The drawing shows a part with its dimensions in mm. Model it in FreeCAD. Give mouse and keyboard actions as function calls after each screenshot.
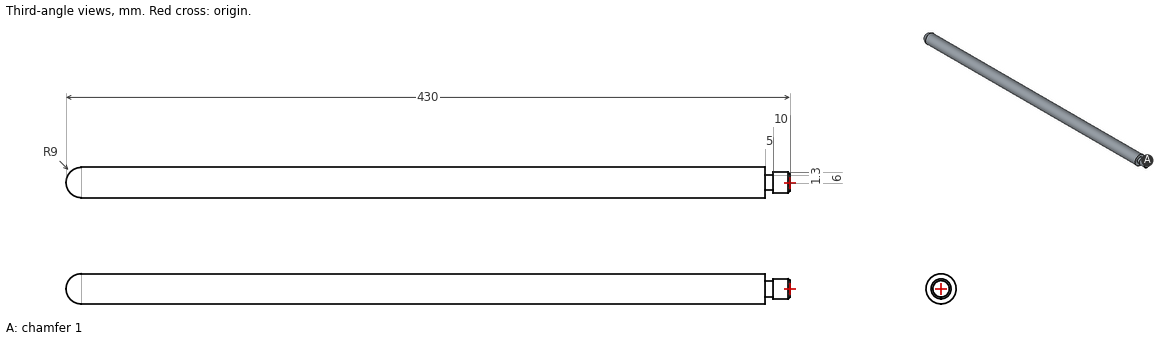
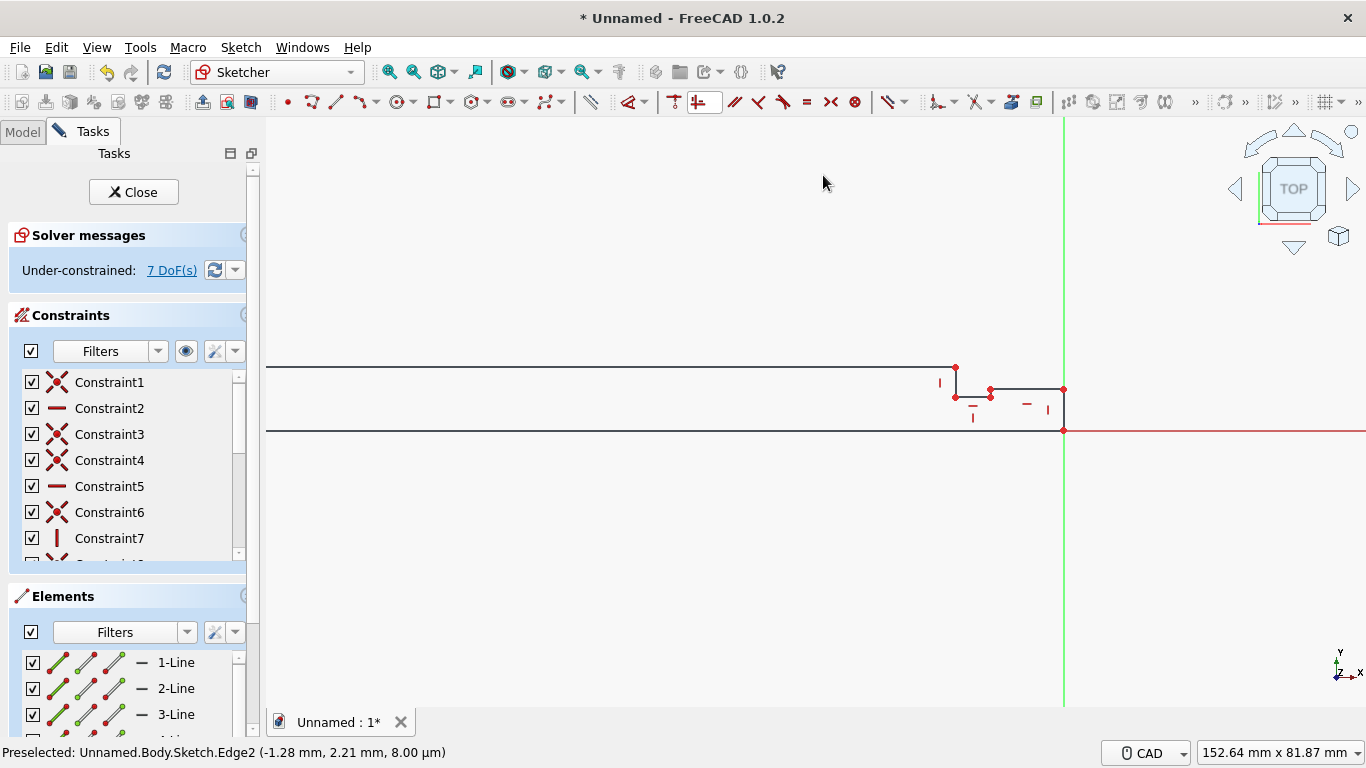
scroll(1059, 415, down, 8)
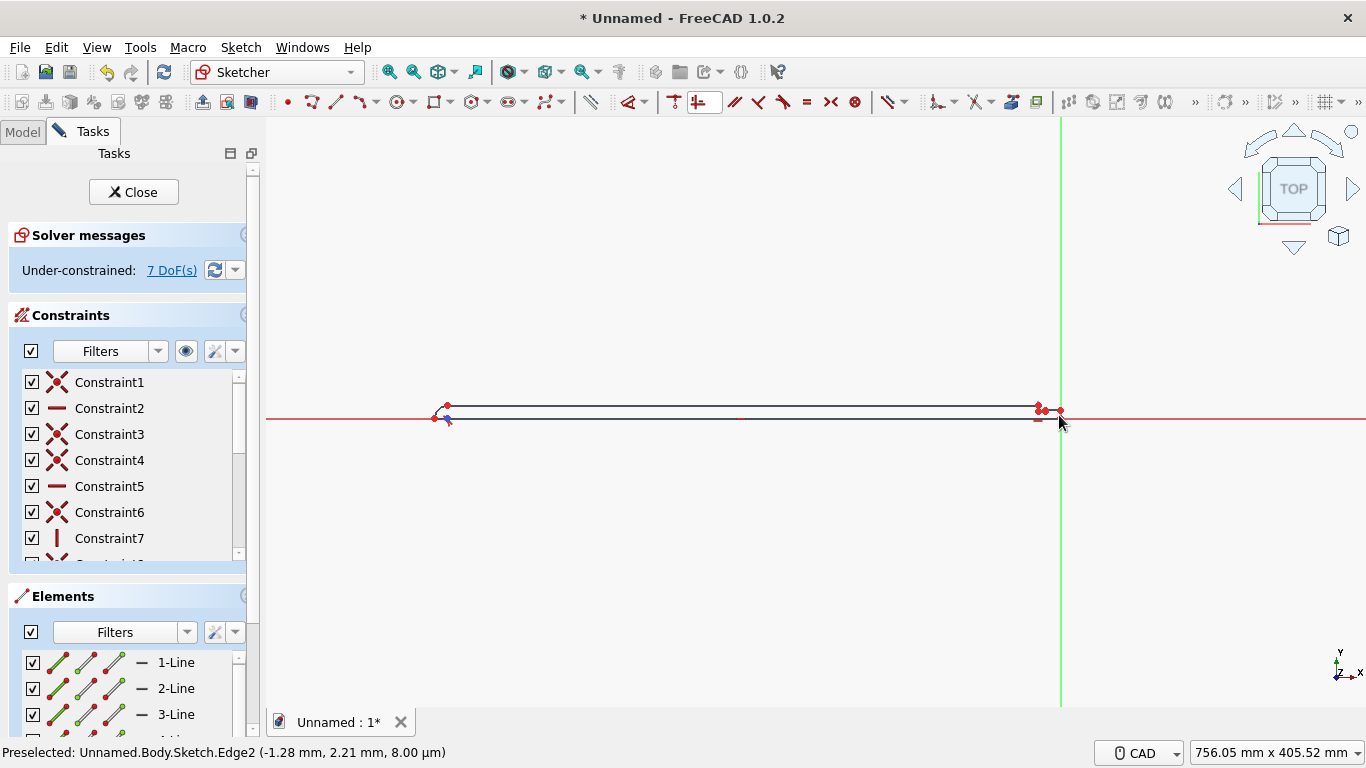
click(448, 419)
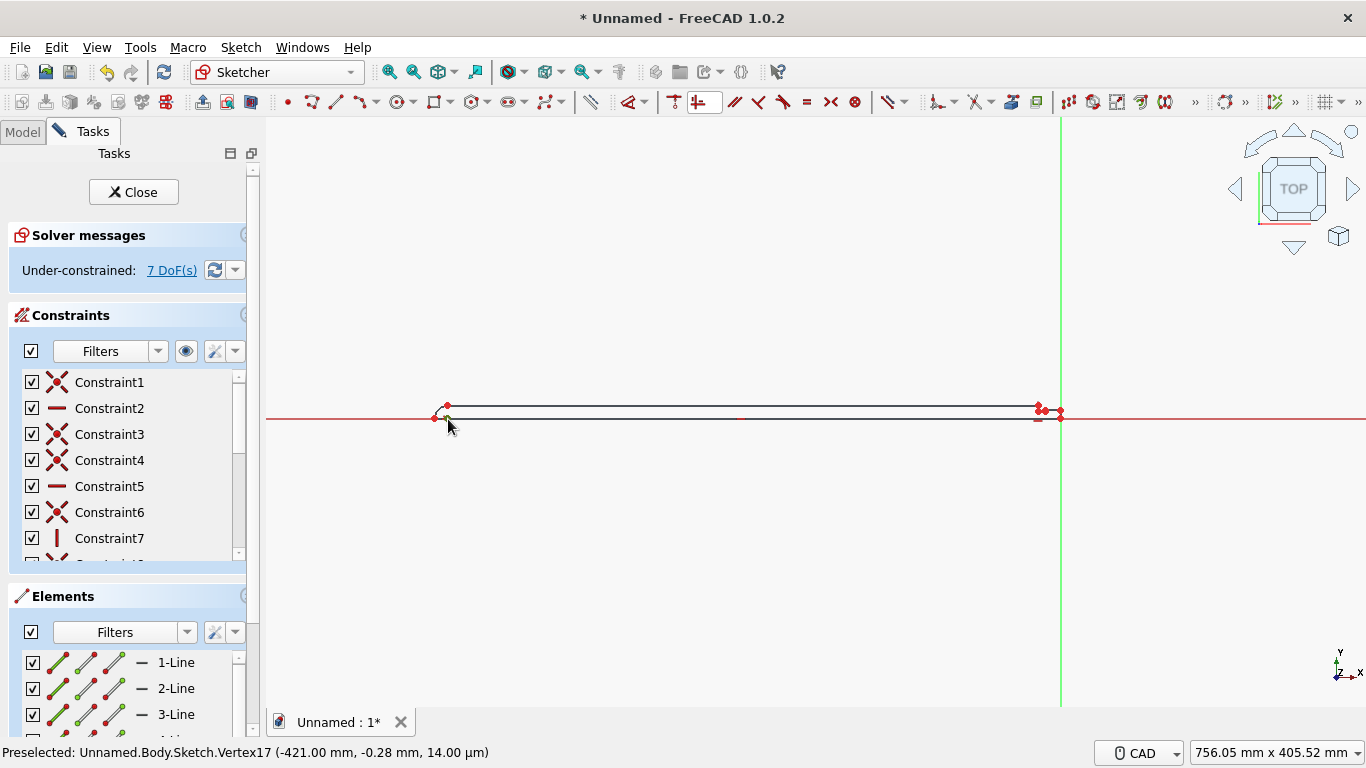
click(359, 419)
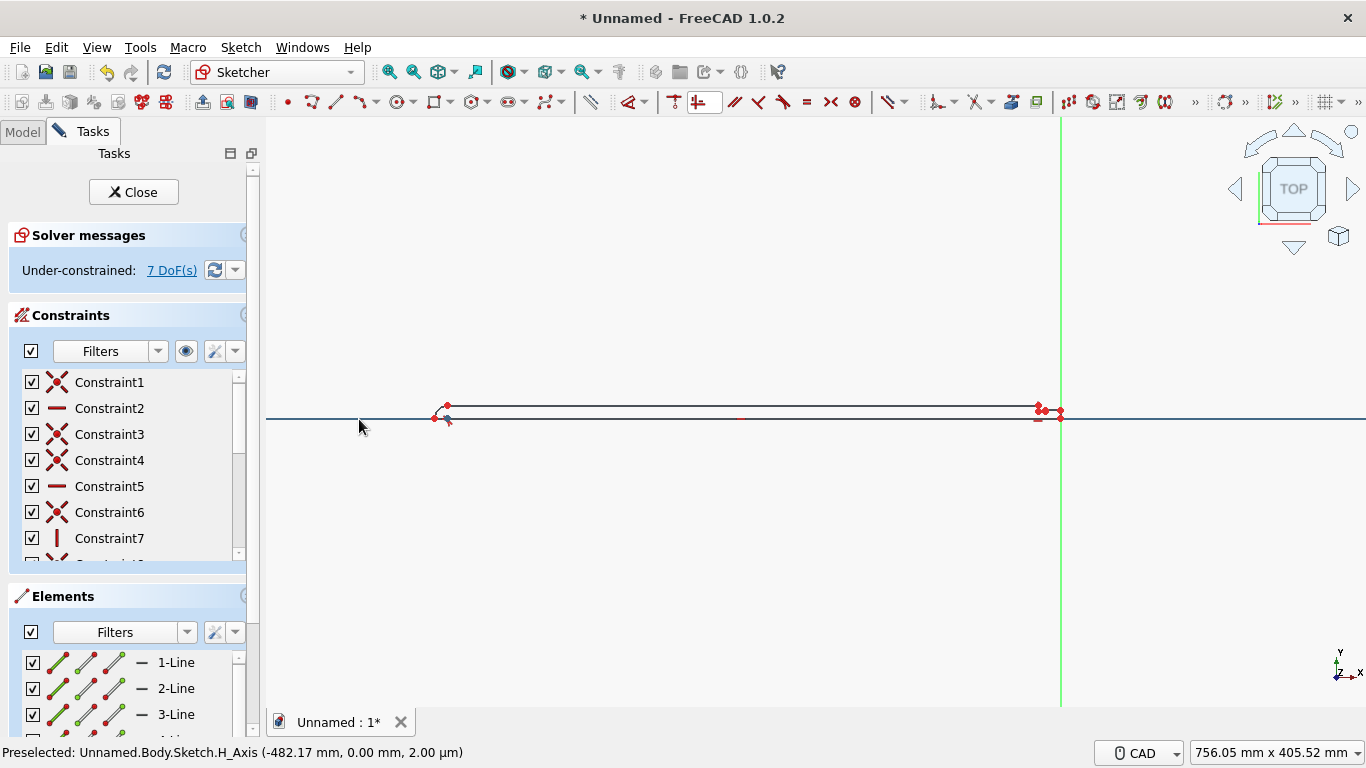
click(674, 102)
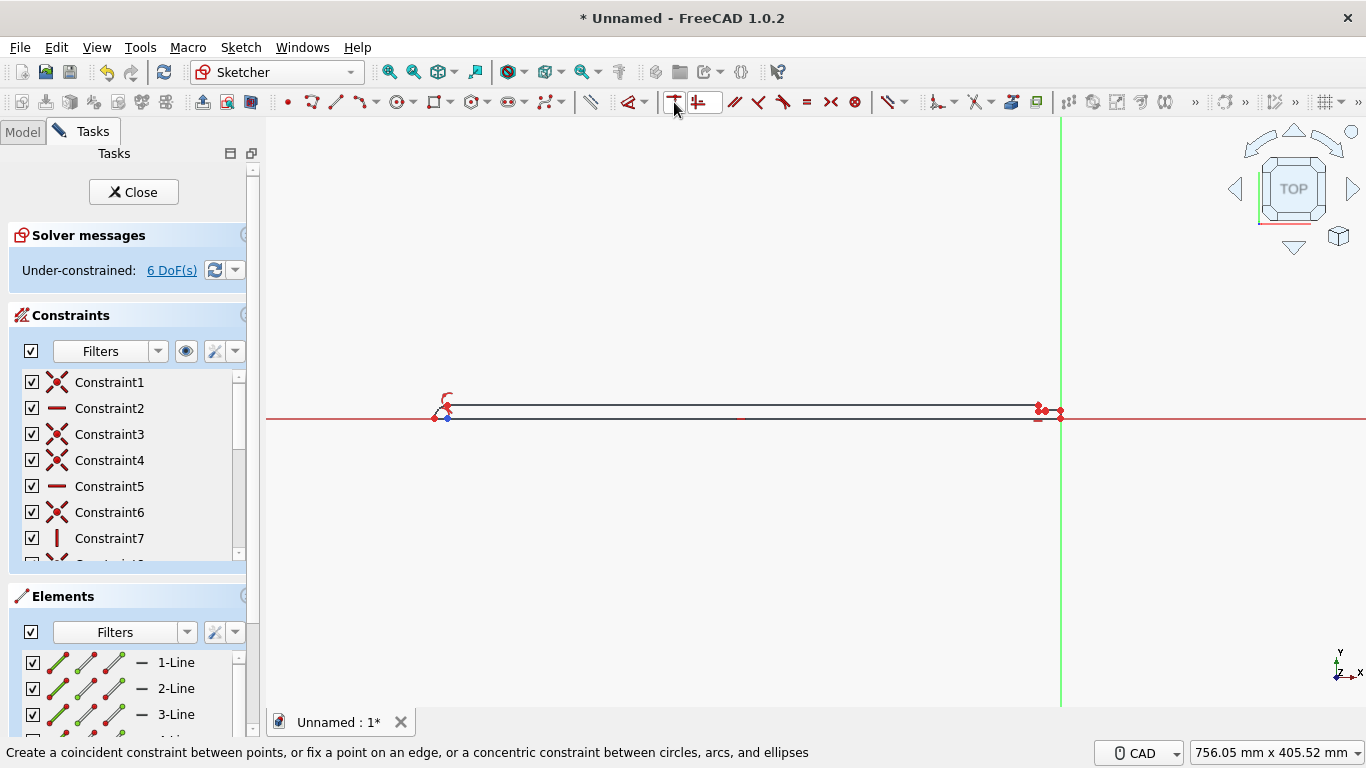
click(628, 102)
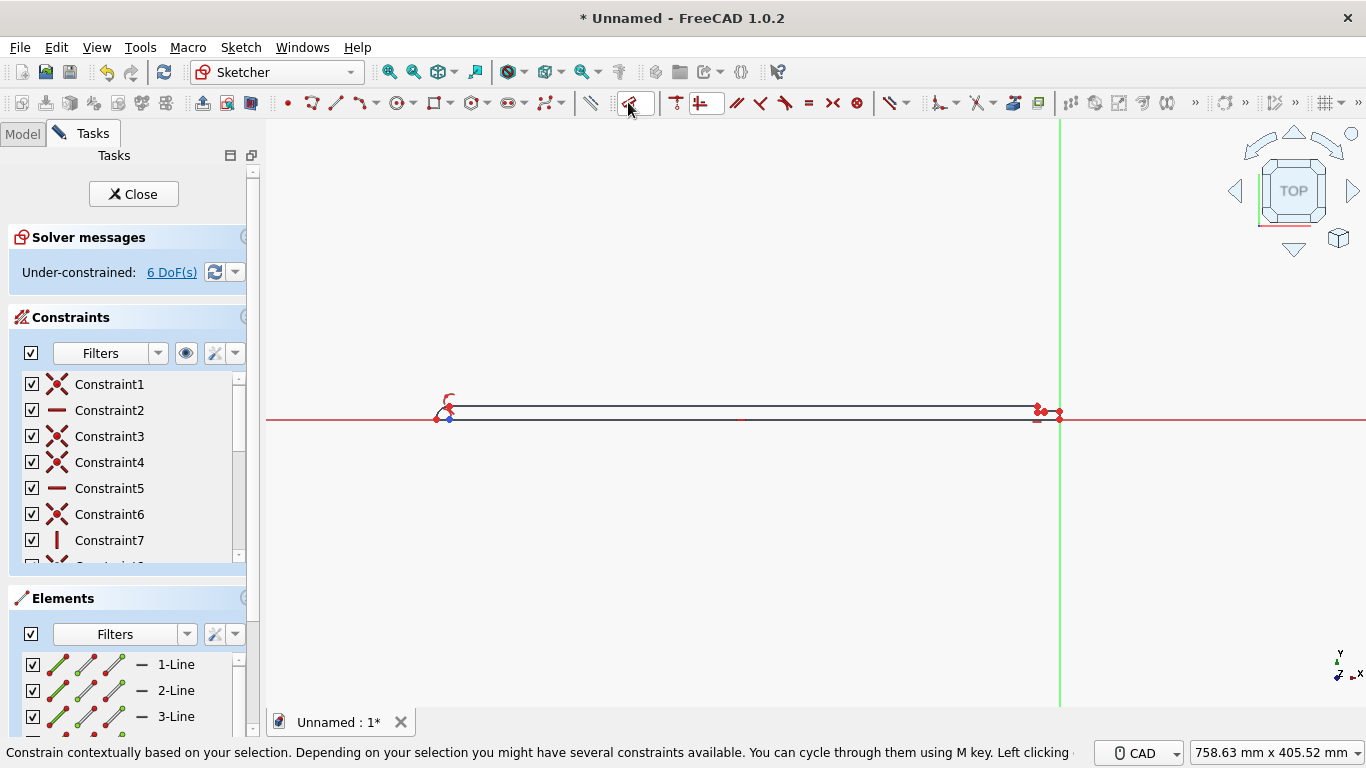
scroll(440, 410, up, 6)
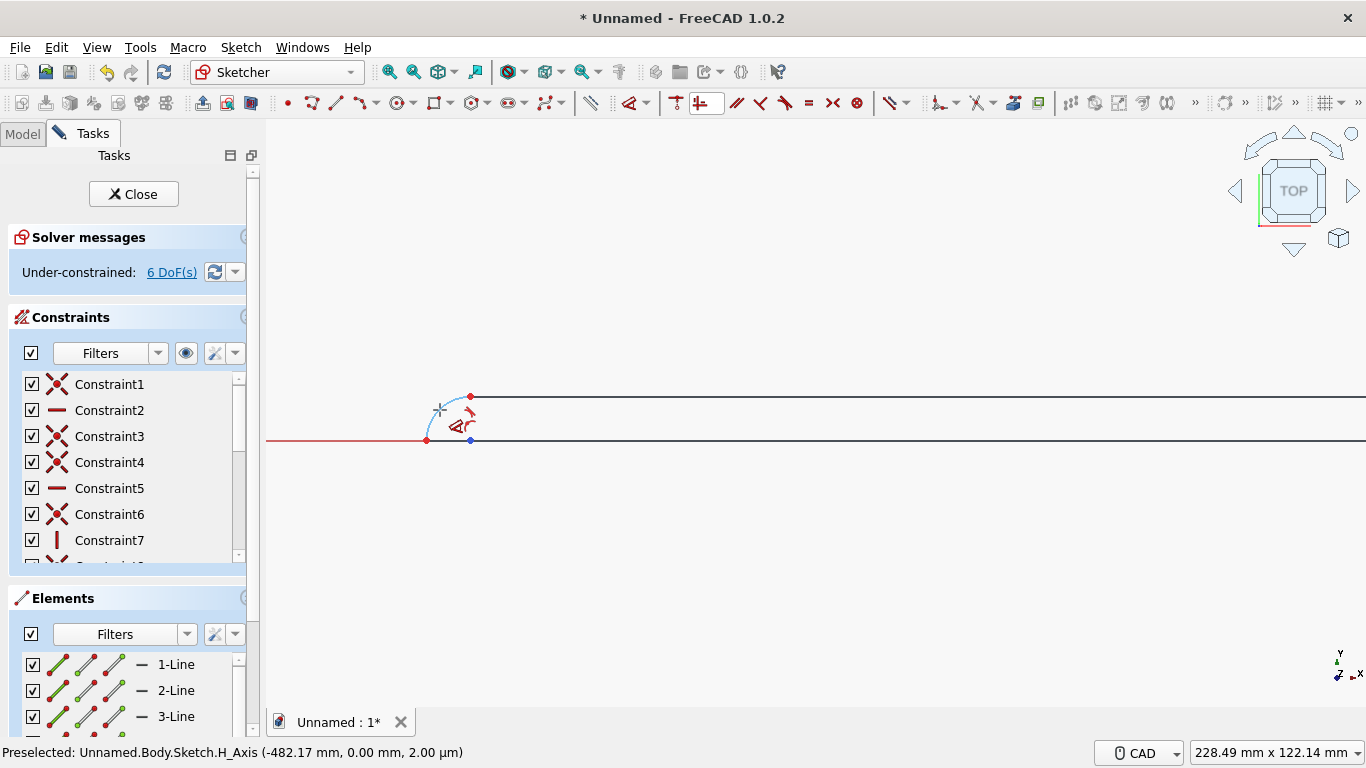
click(439, 410)
click(416, 388)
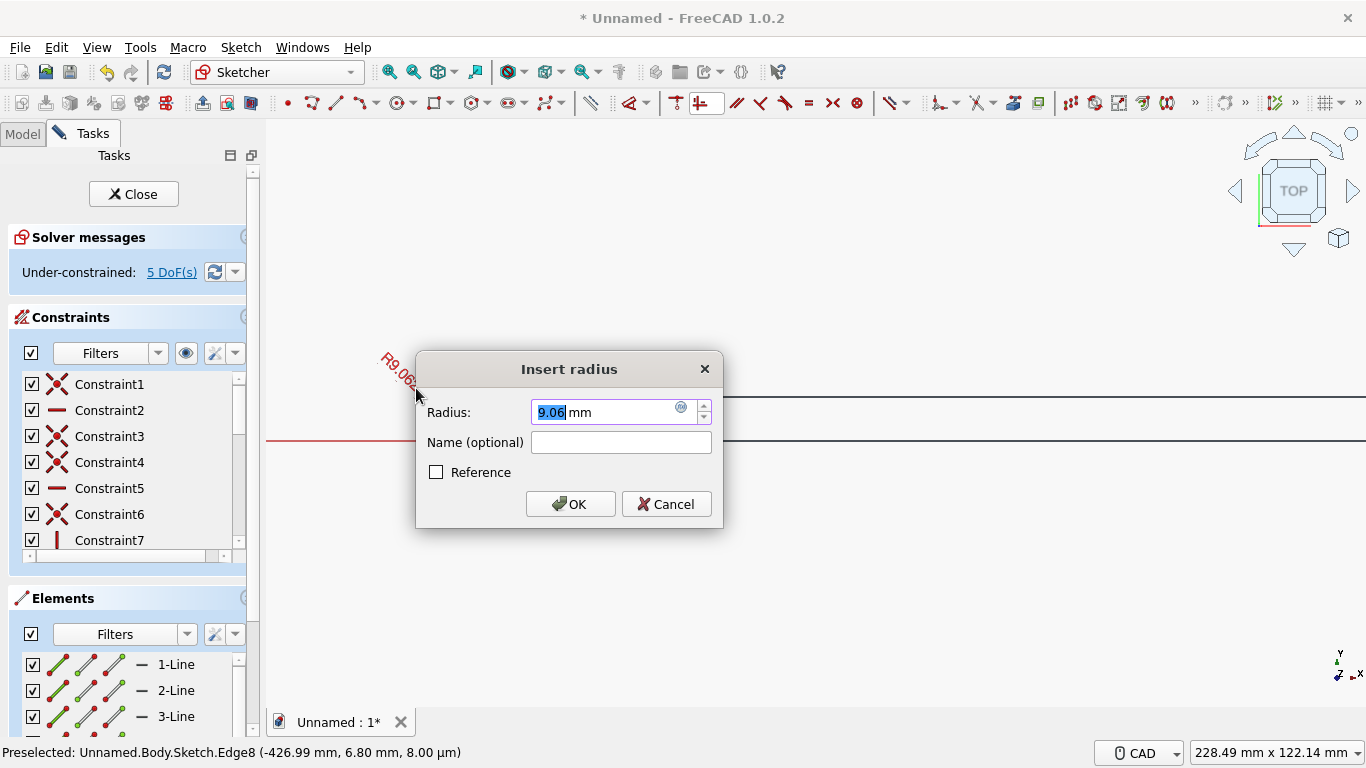
text(9)
key(Return)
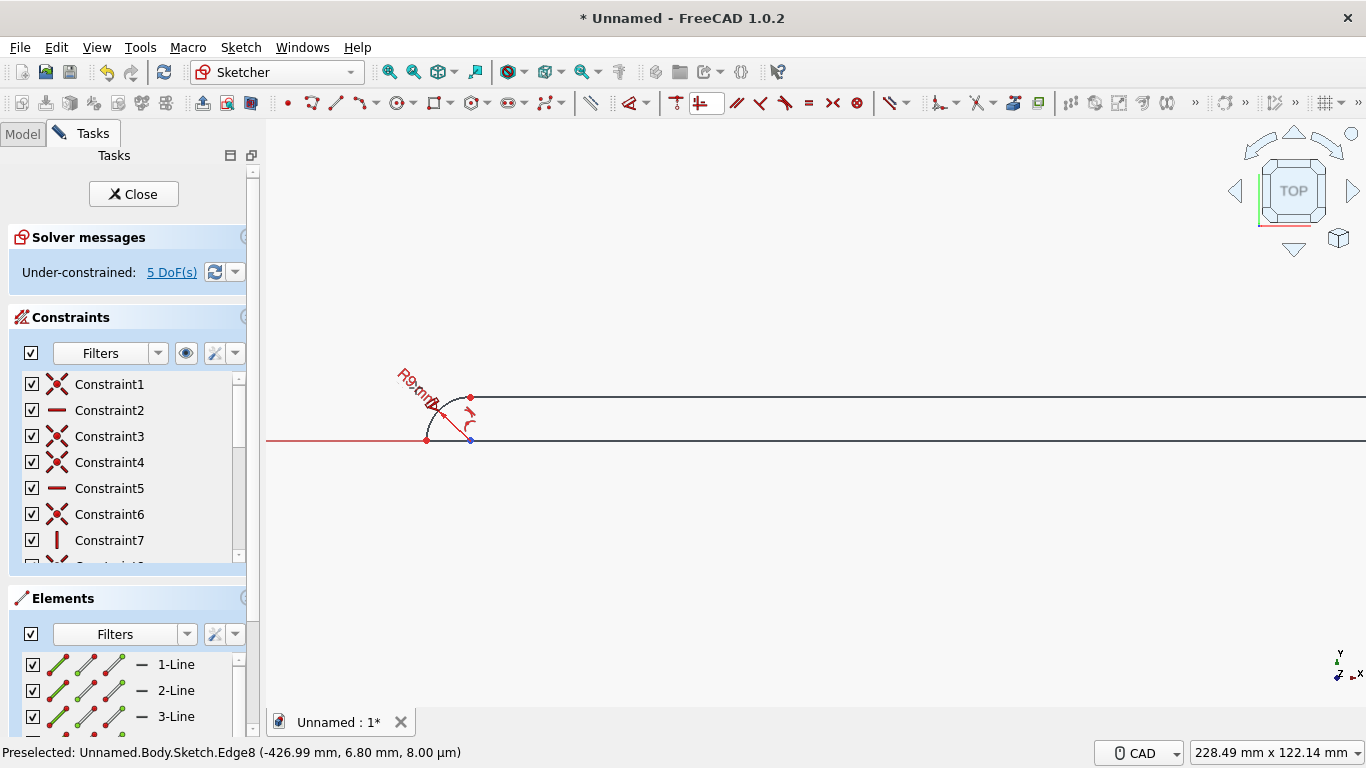
scroll(440, 410, down, 6)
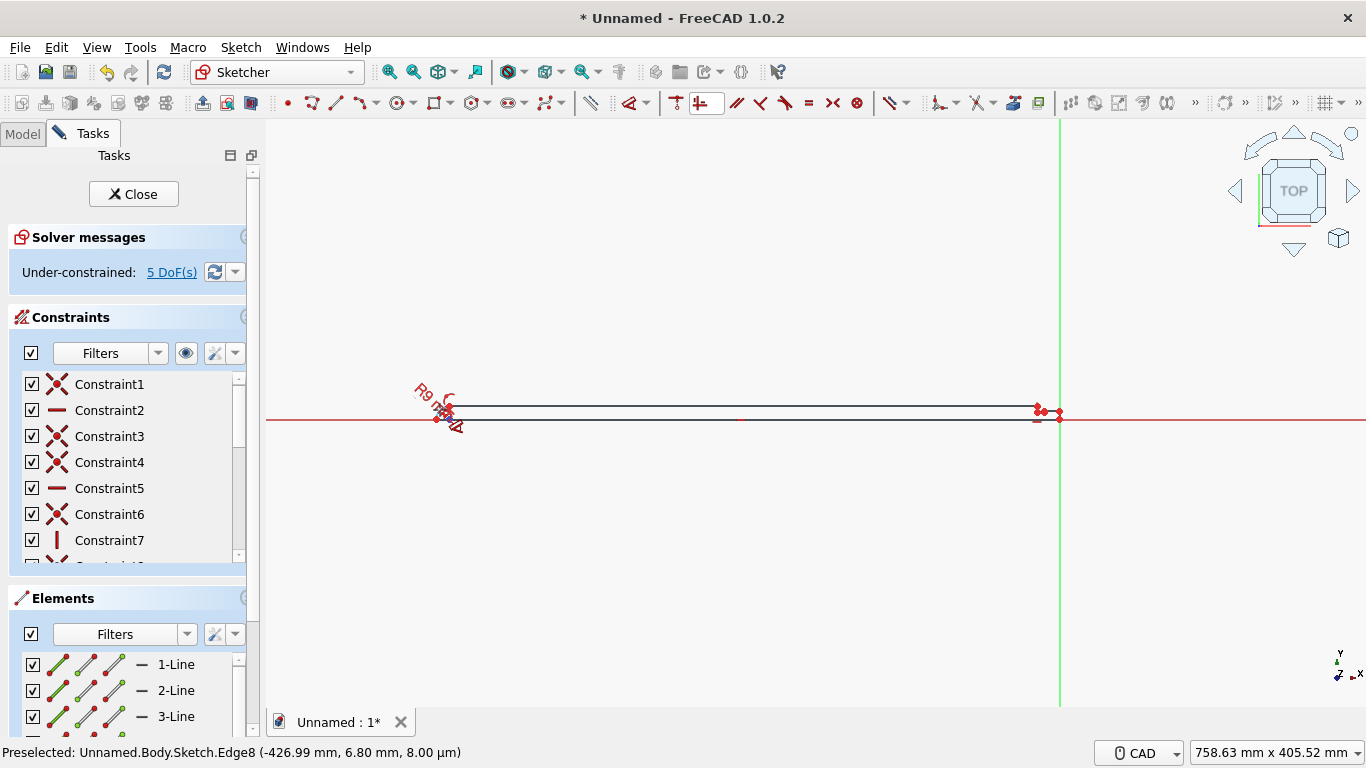
scroll(1060, 416, up, 8)